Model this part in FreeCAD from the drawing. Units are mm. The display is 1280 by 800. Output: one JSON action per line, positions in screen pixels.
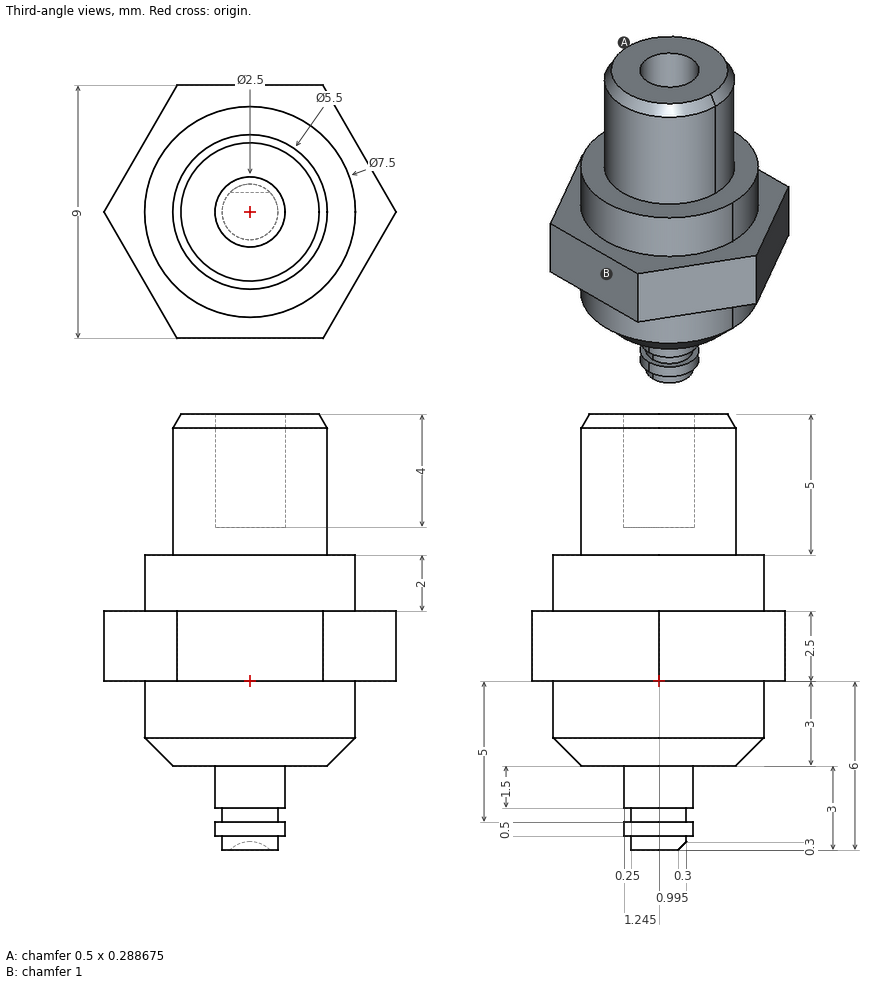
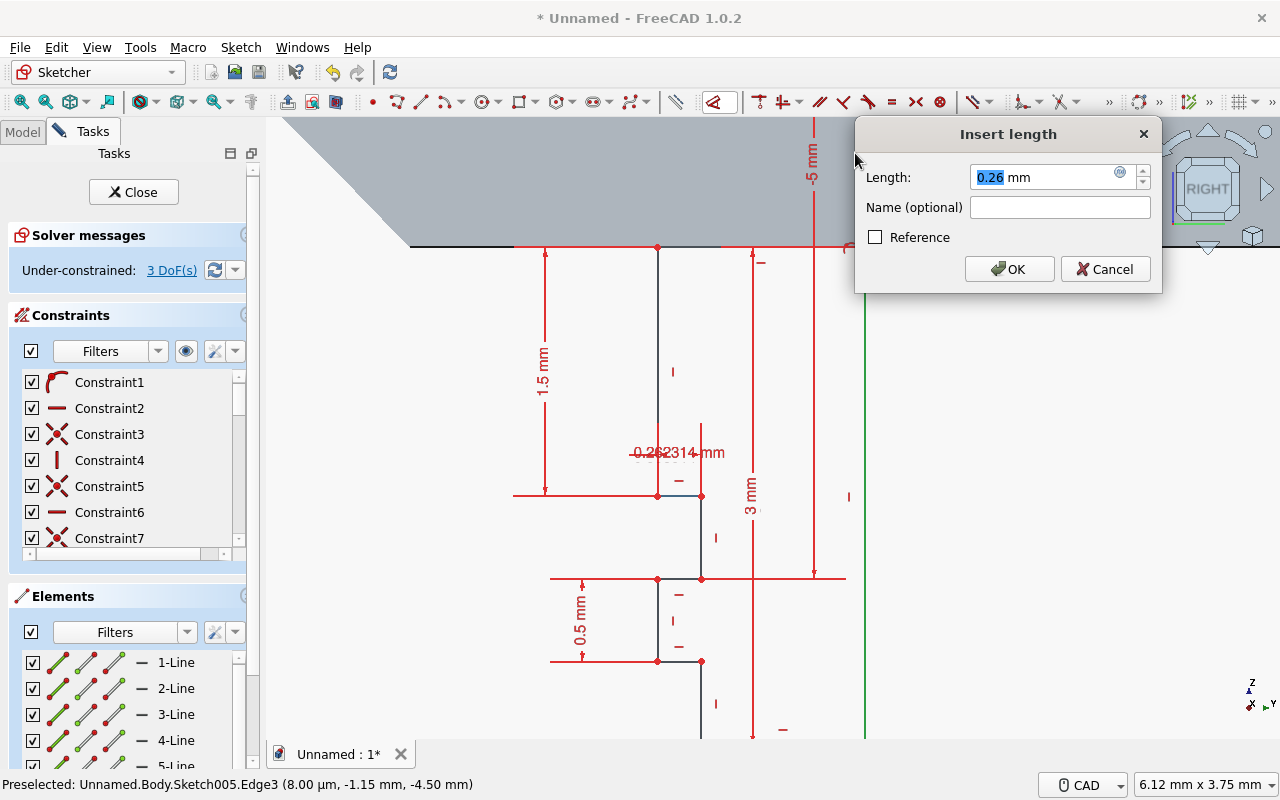
{"action": "type", "text": "0.25"}
{"action": "key", "text": "Return"}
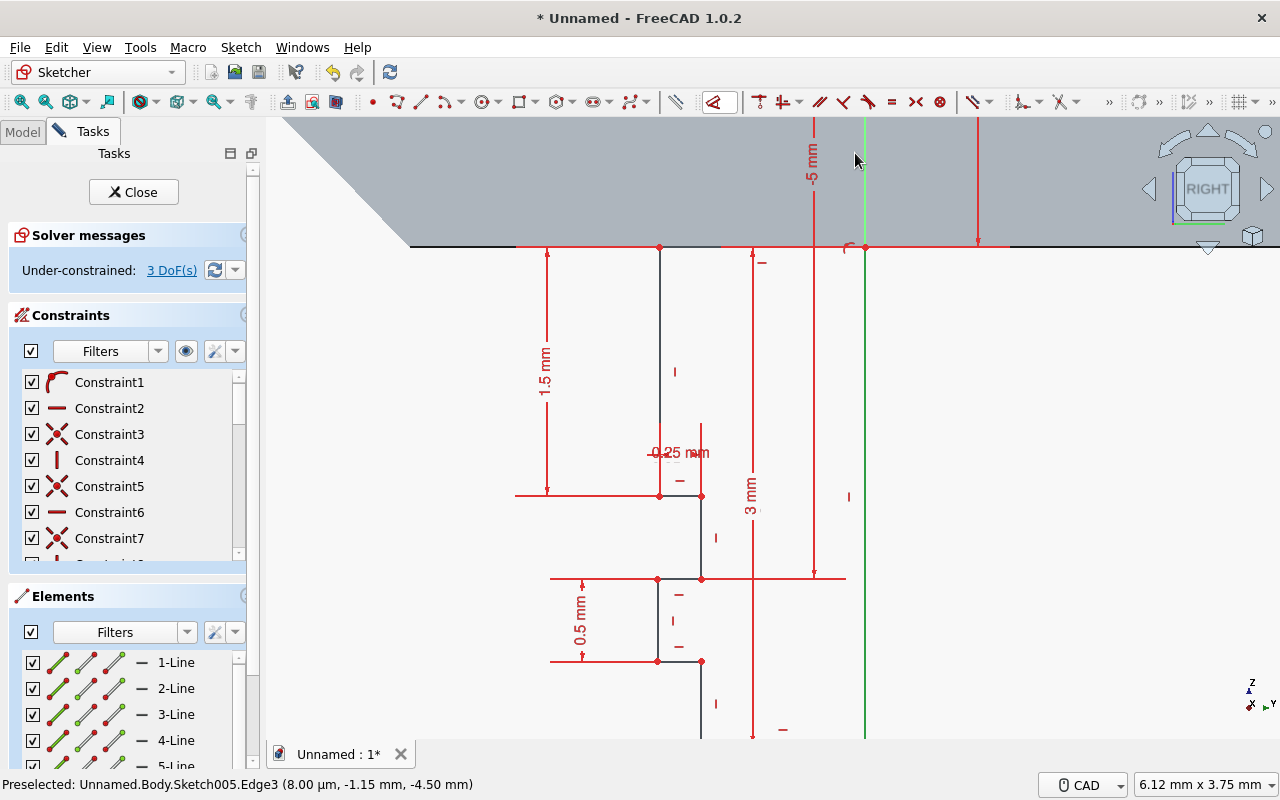
{"action": "left_click", "coordinate": [688, 579]}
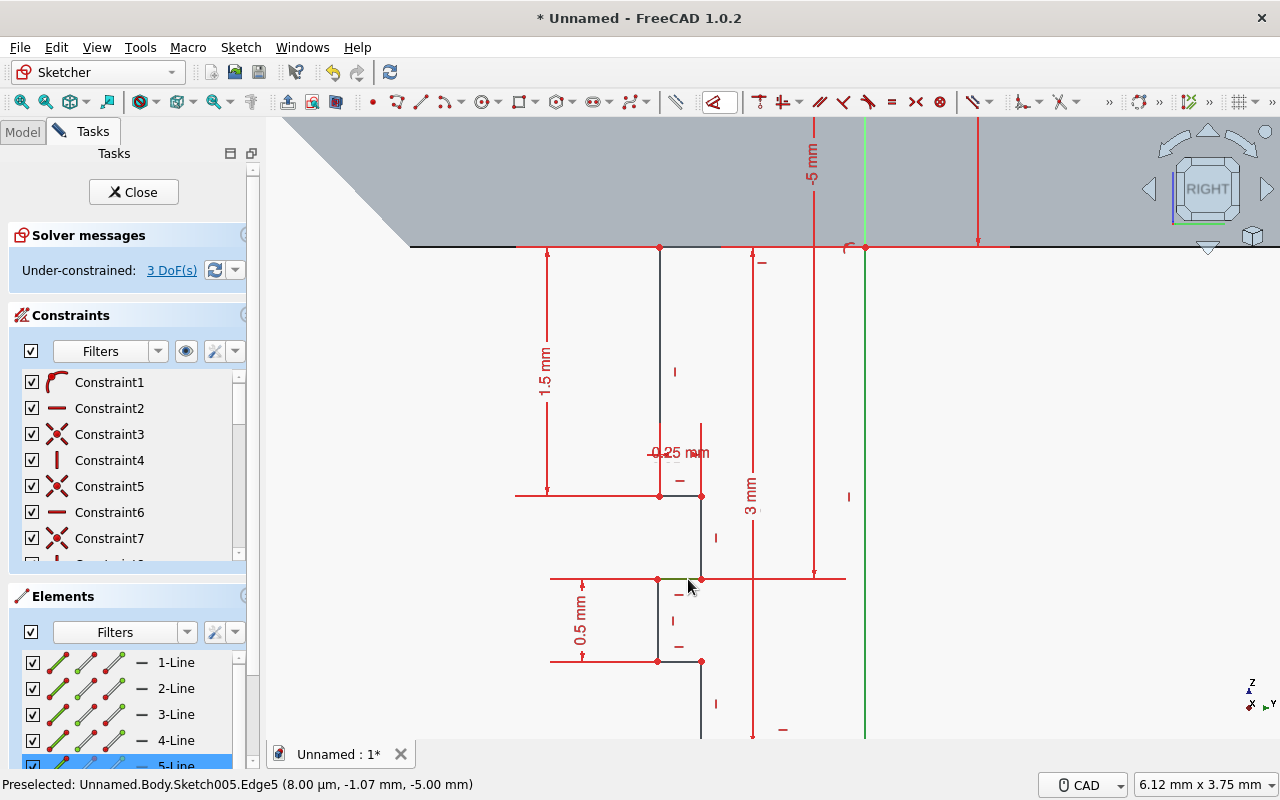
{"action": "key", "text": "l"}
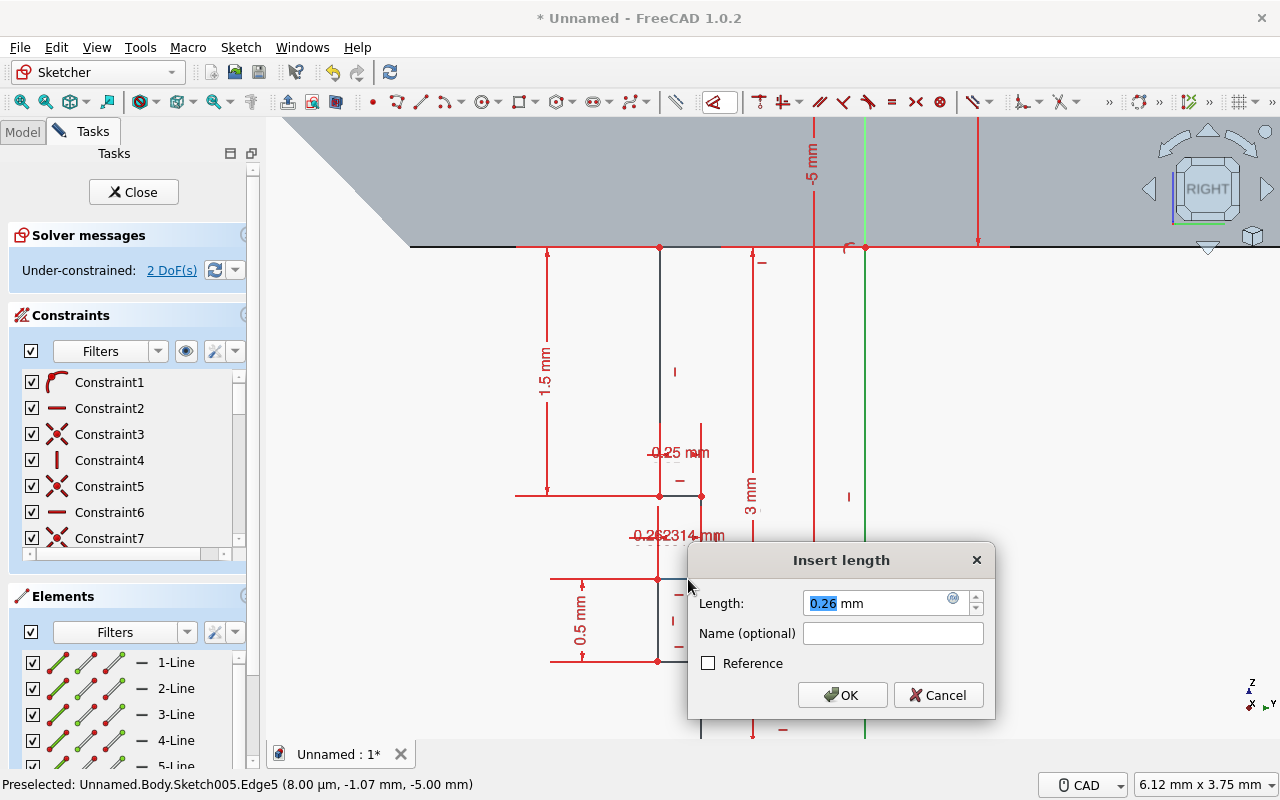
{"action": "type", "text": "0.25"}
{"action": "key", "text": "Return"}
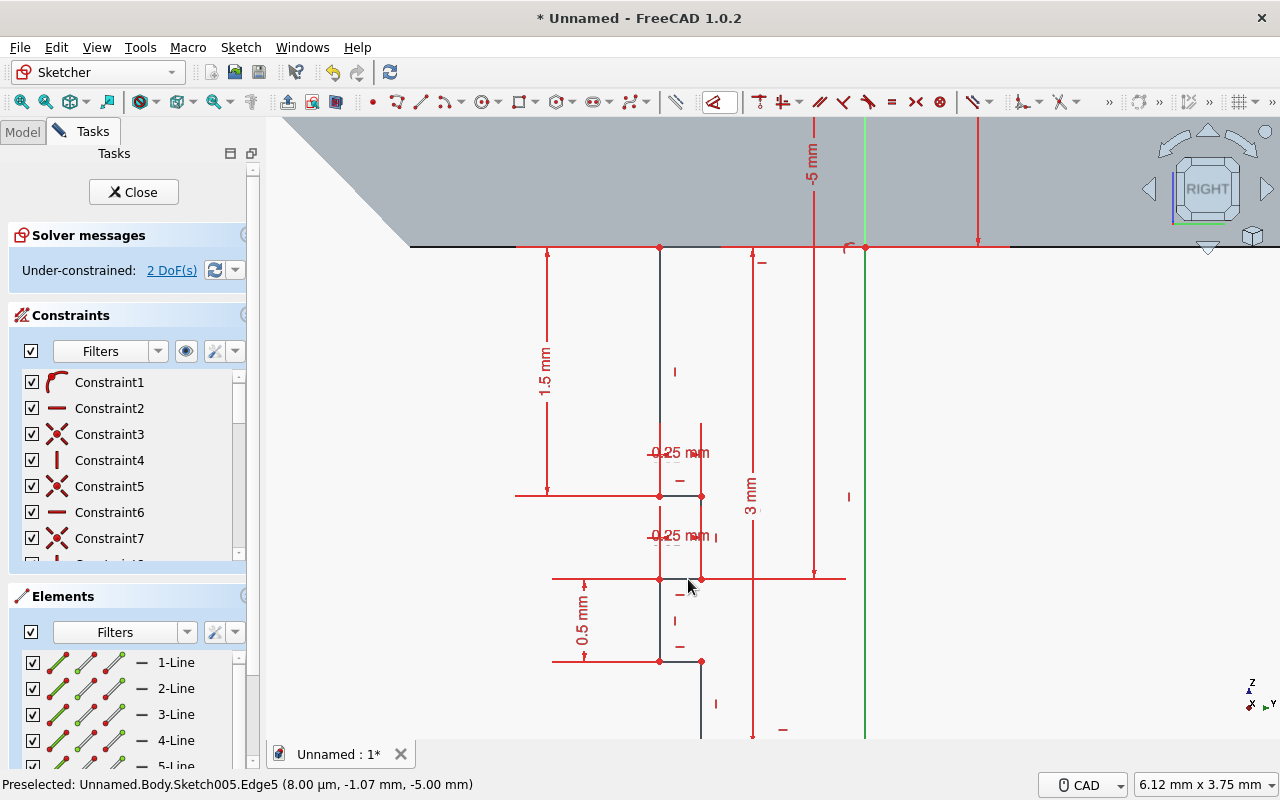
{"action": "left_click", "coordinate": [672, 662]}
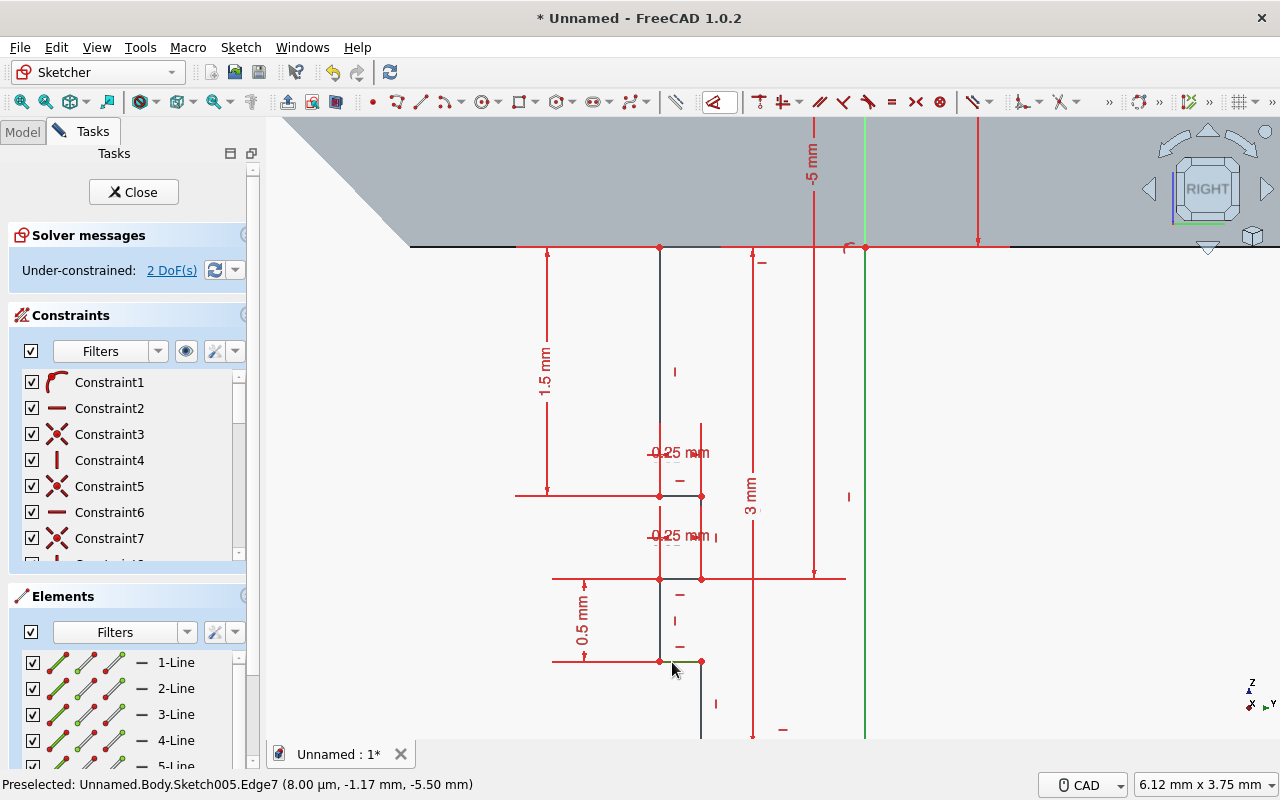
{"action": "left_click", "coordinate": [732, 102]}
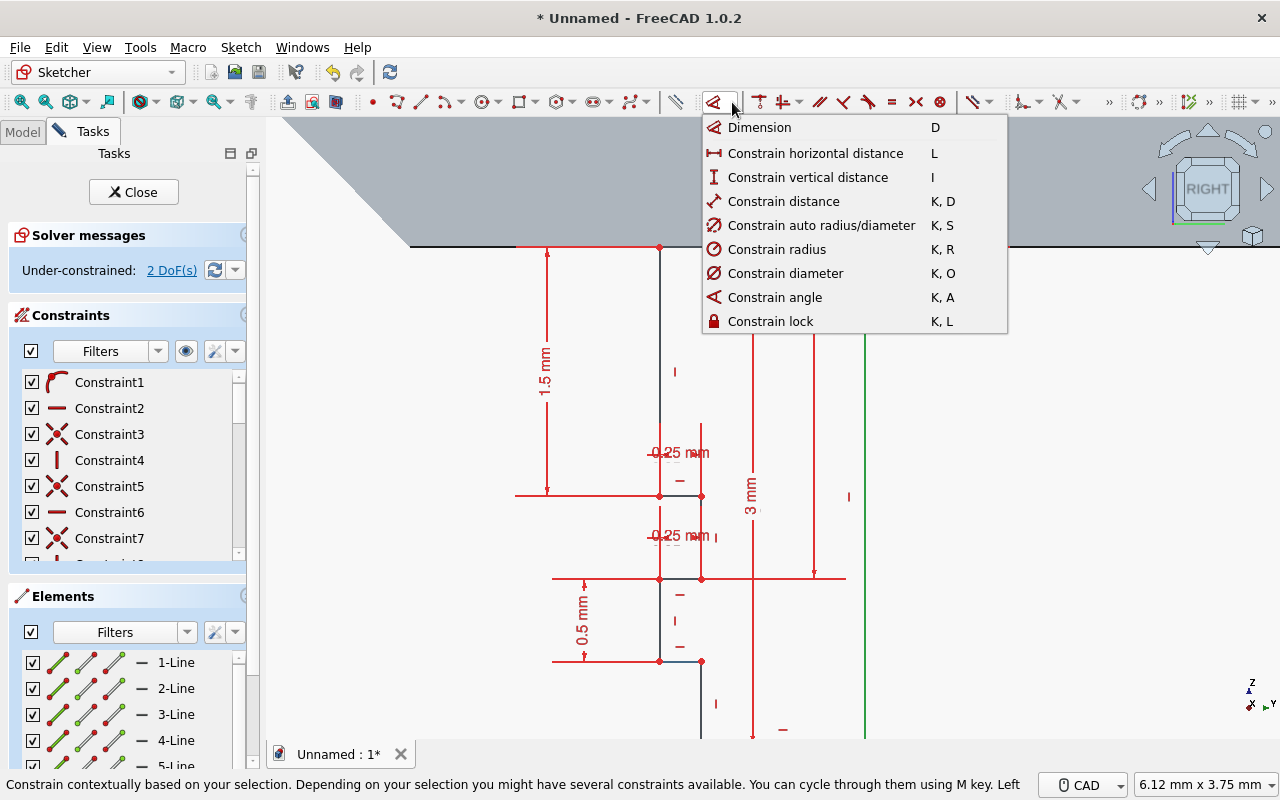
{"action": "left_click", "coordinate": [855, 153]}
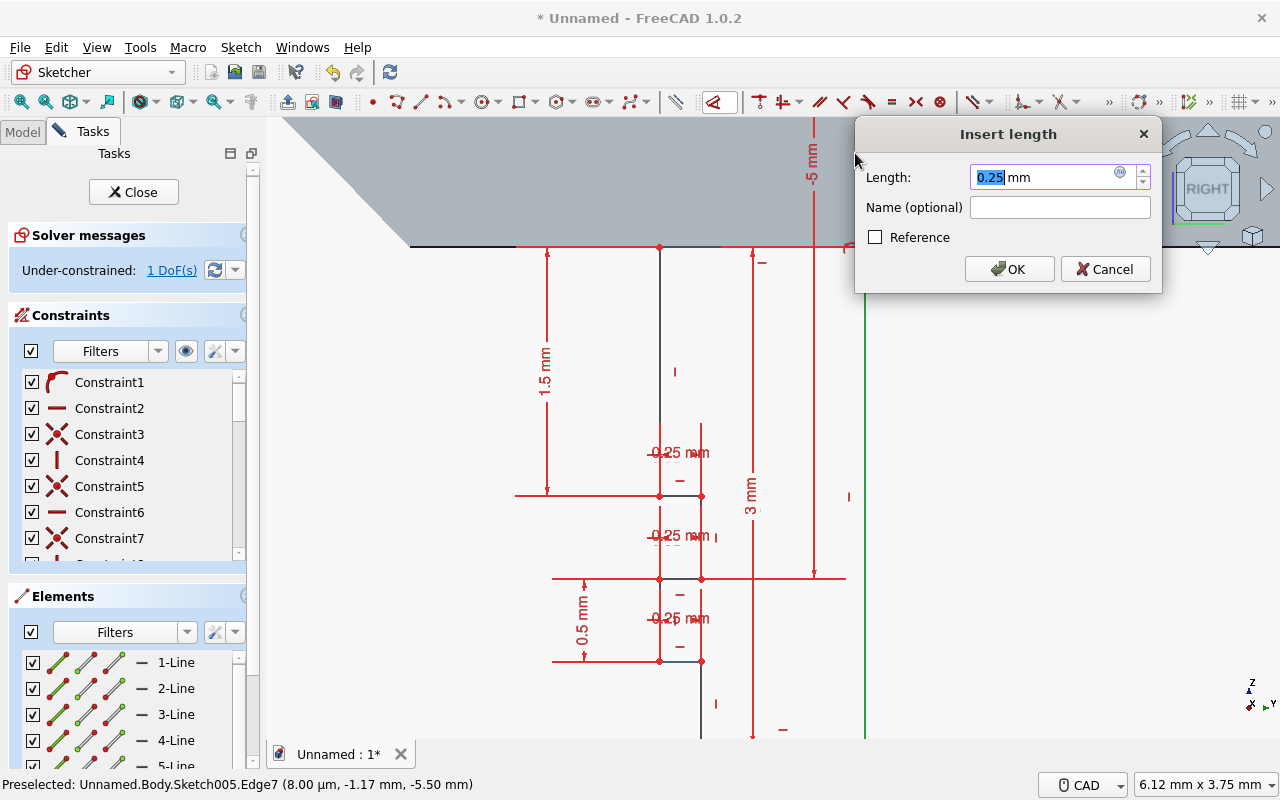
{"action": "type", "text": "0.25"}
{"action": "key", "text": "Return"}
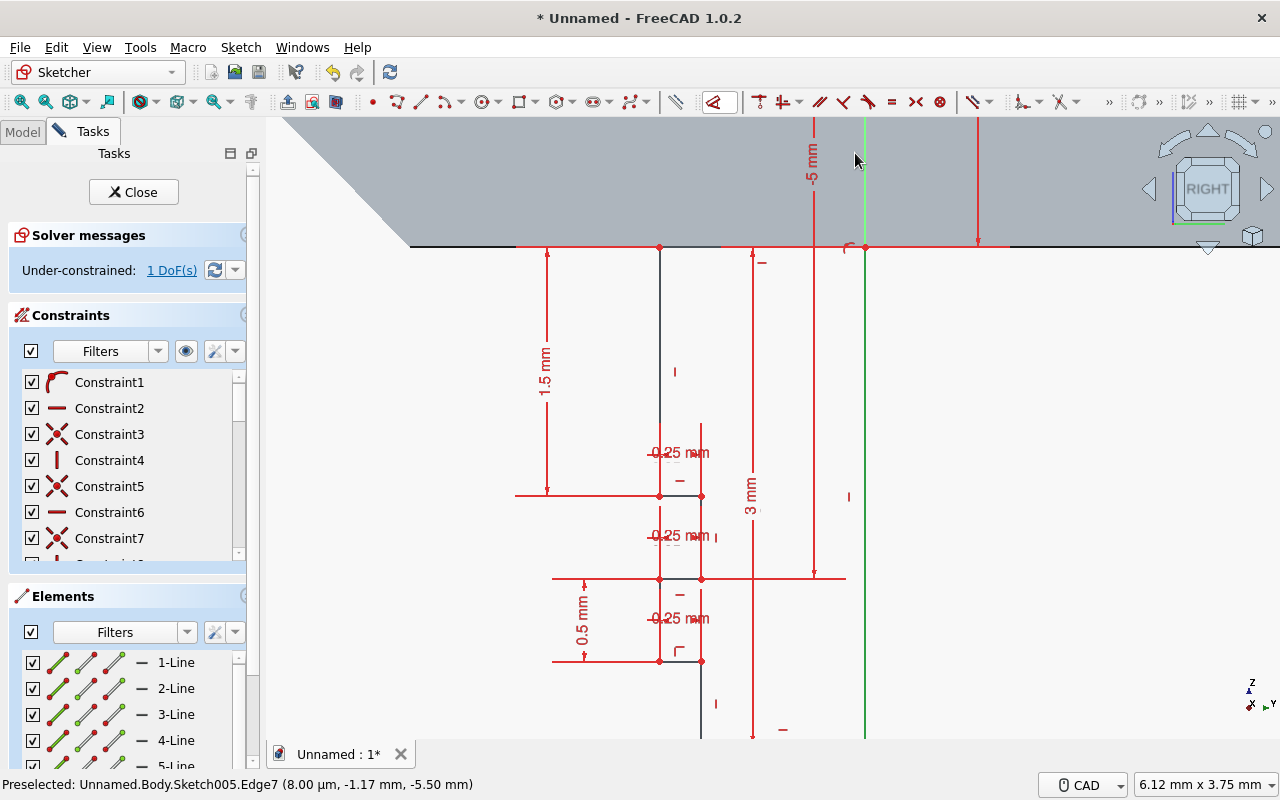
{"action": "left_click", "coordinate": [804, 247]}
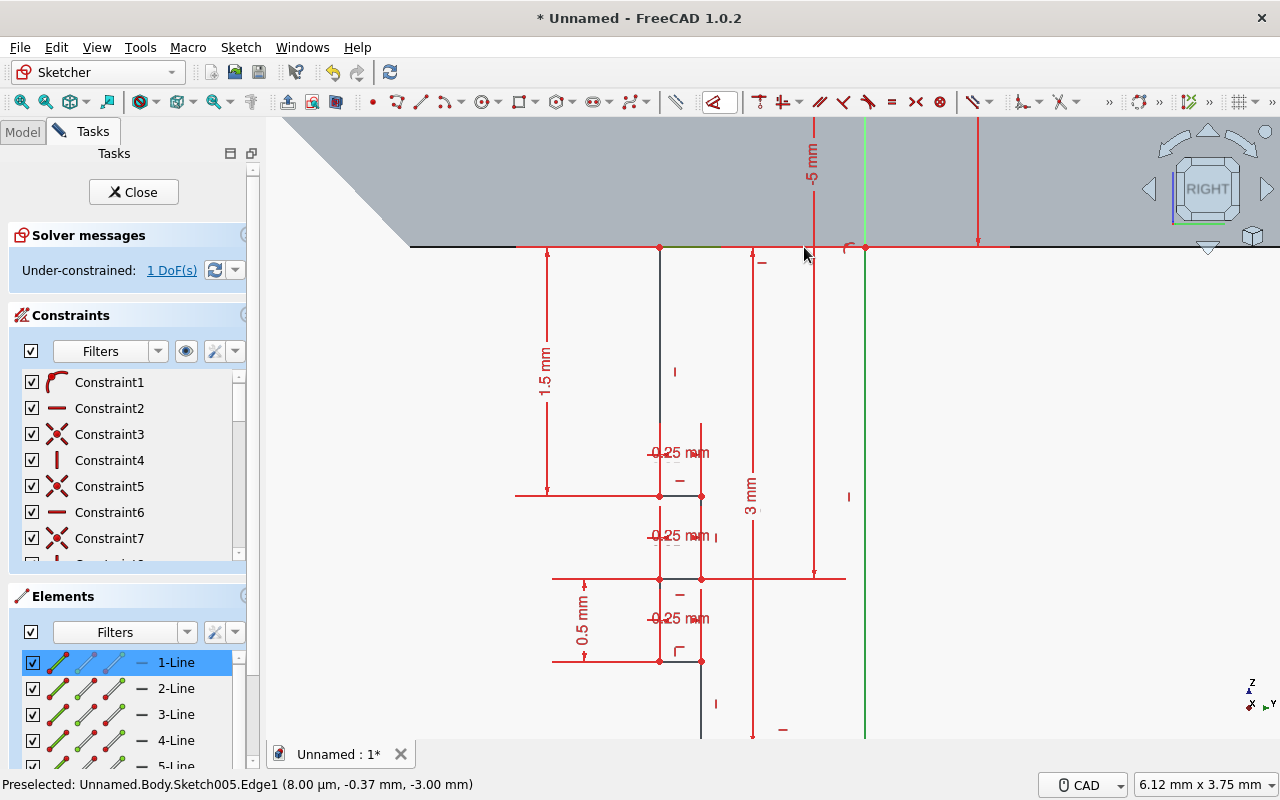
{"action": "key", "text": "l"}